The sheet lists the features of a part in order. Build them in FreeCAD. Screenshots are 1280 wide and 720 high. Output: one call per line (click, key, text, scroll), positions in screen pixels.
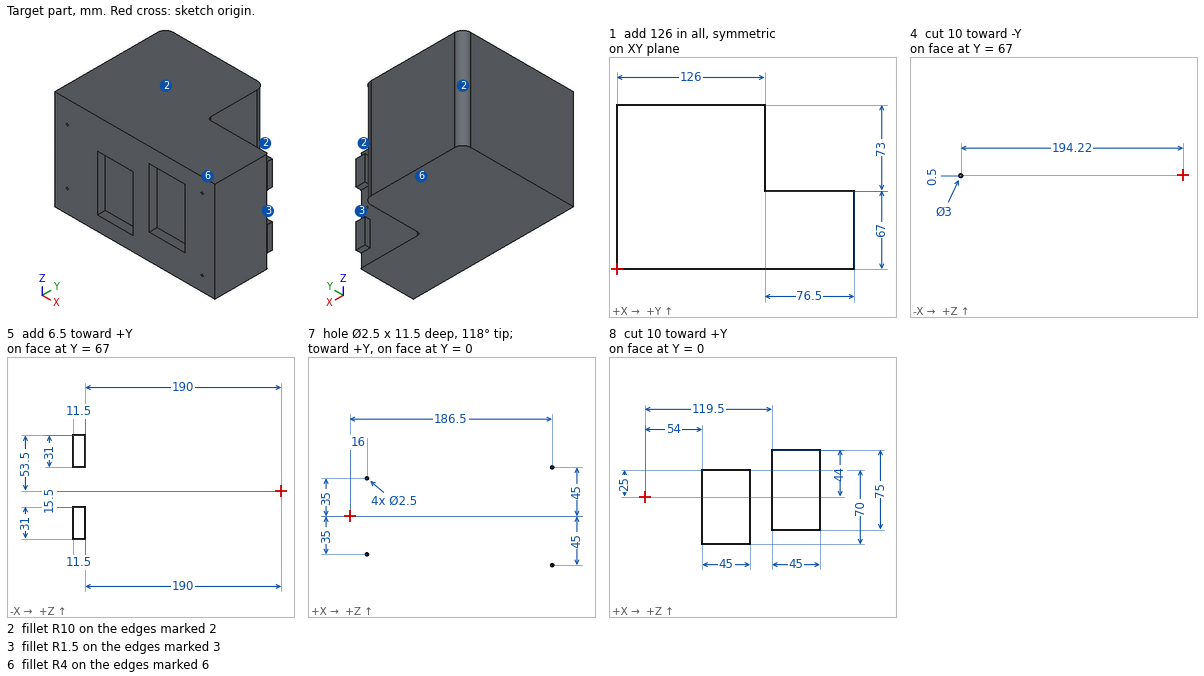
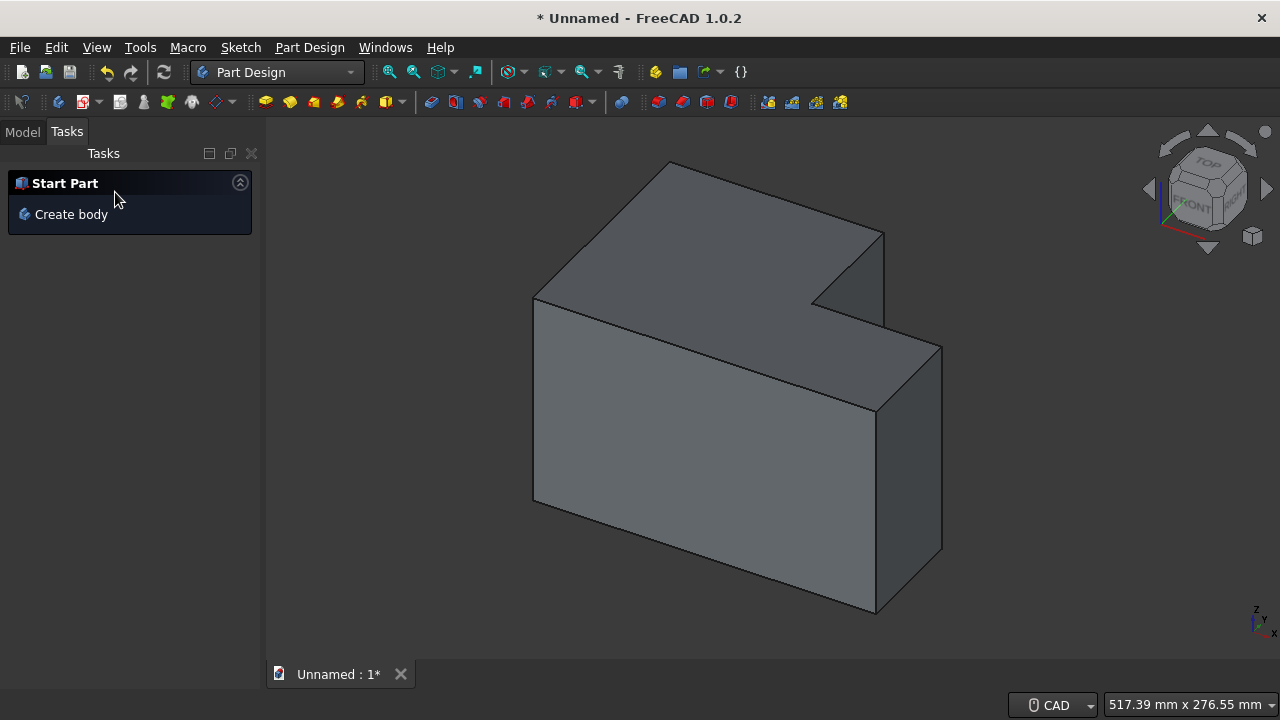
key(0)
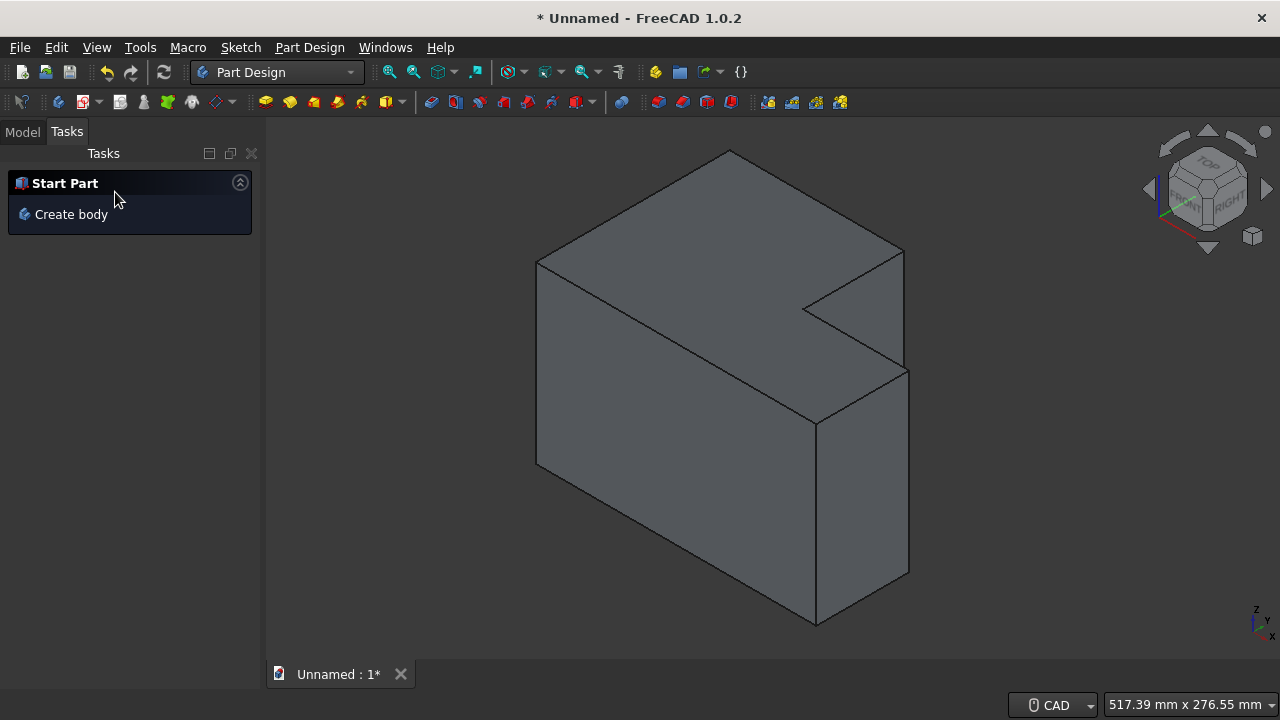
key(2)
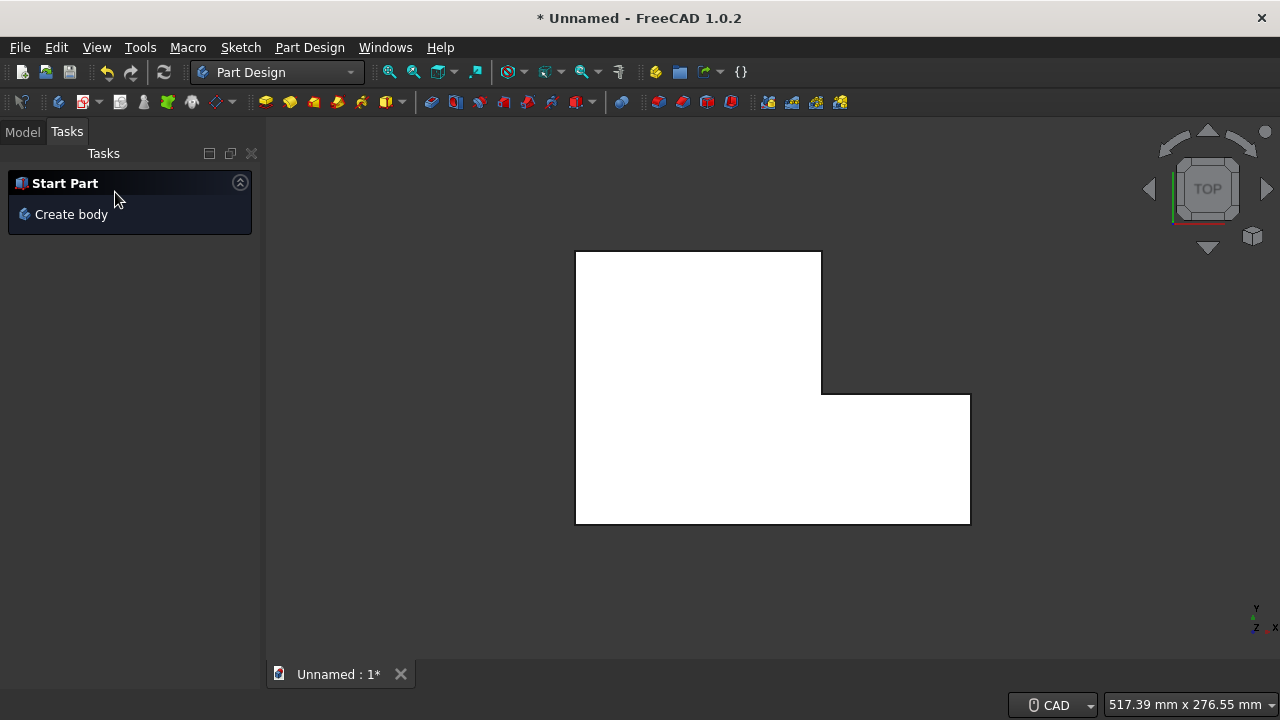
key(1)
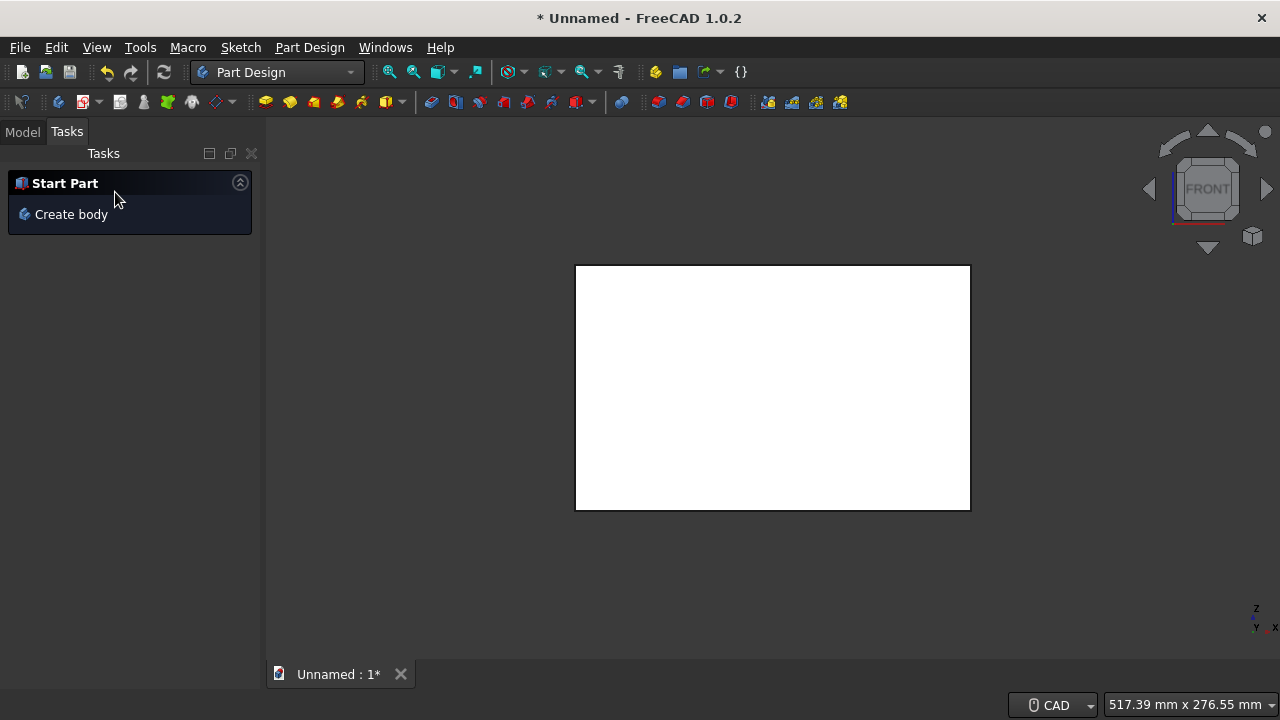
key(3)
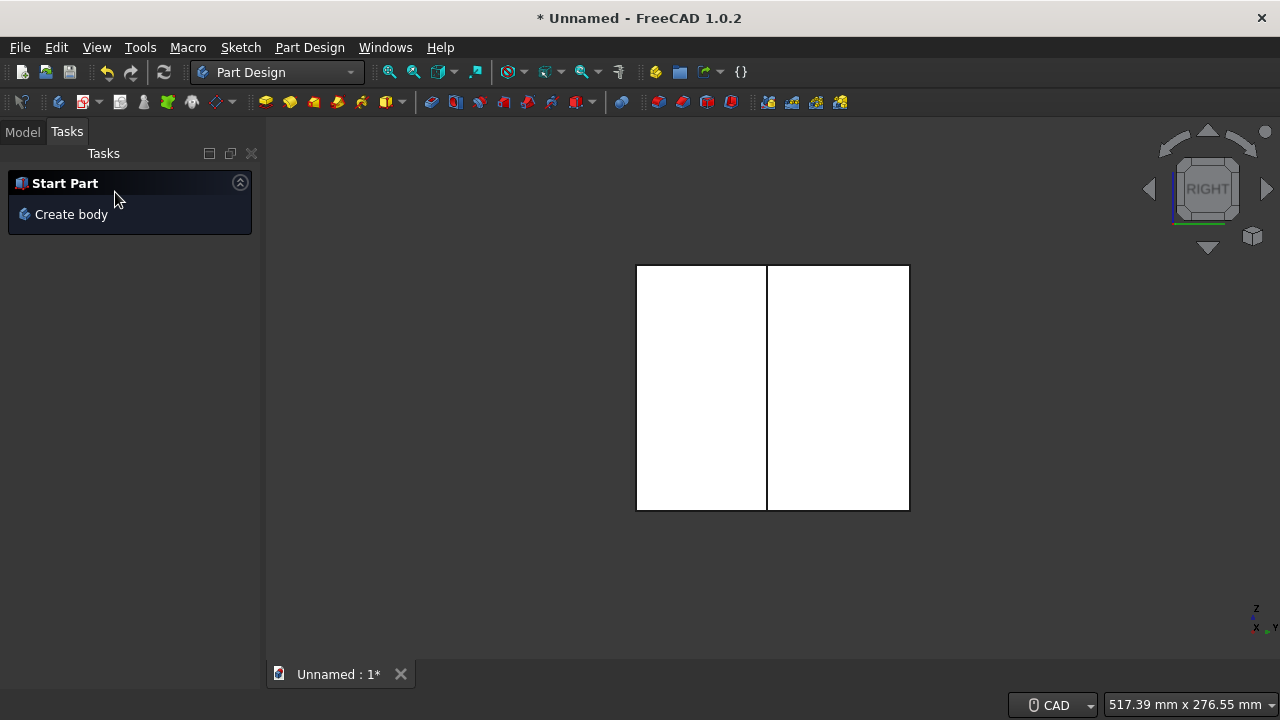
click(910, 387)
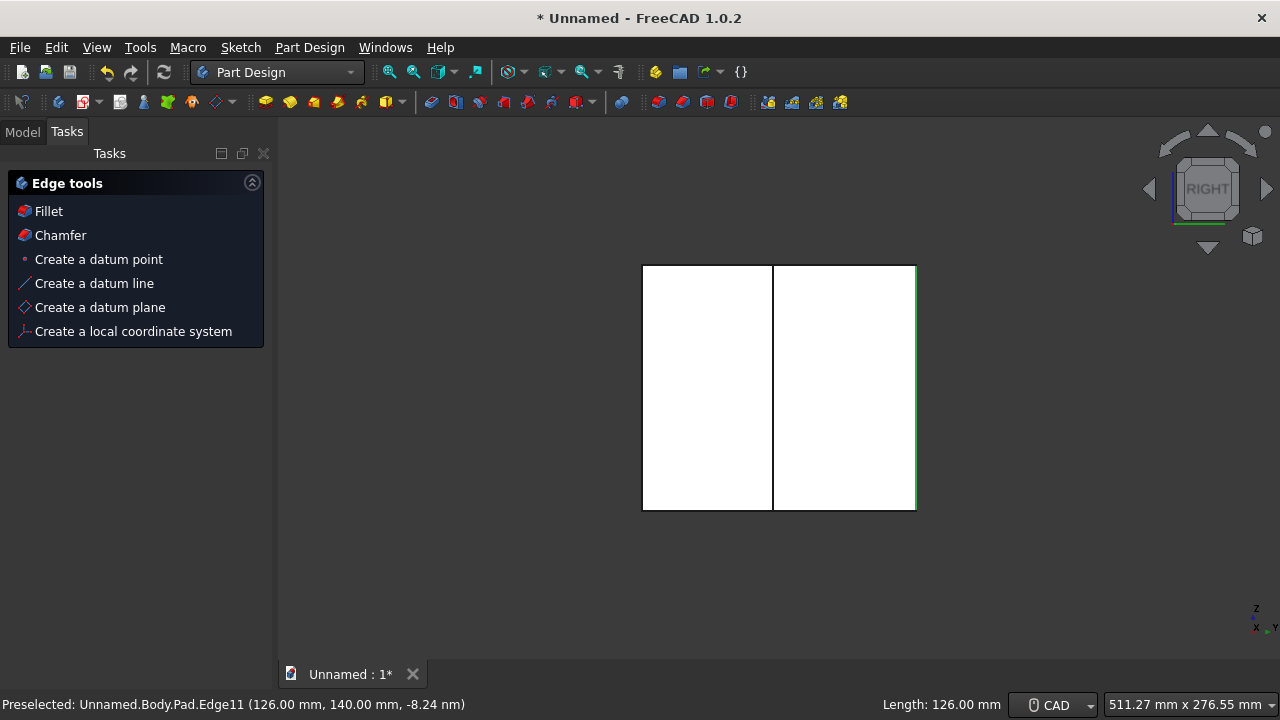
key(5)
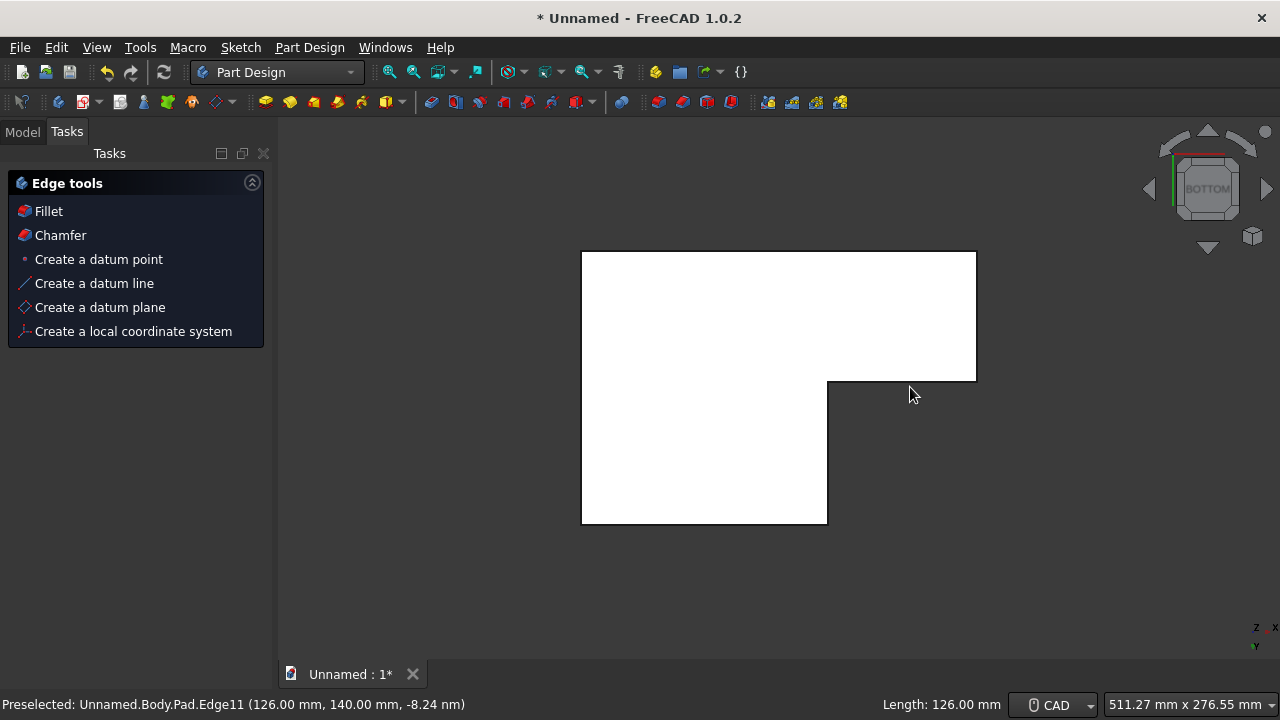
key(4)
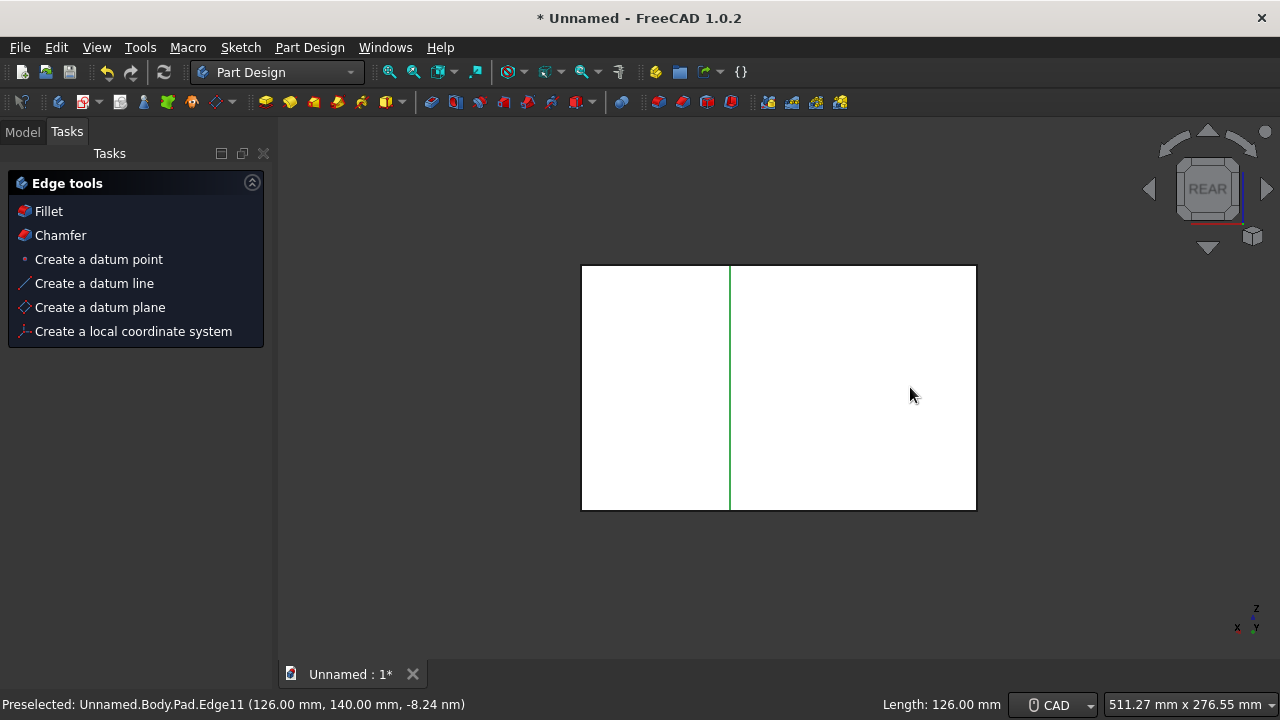
click(977, 387, ctrl)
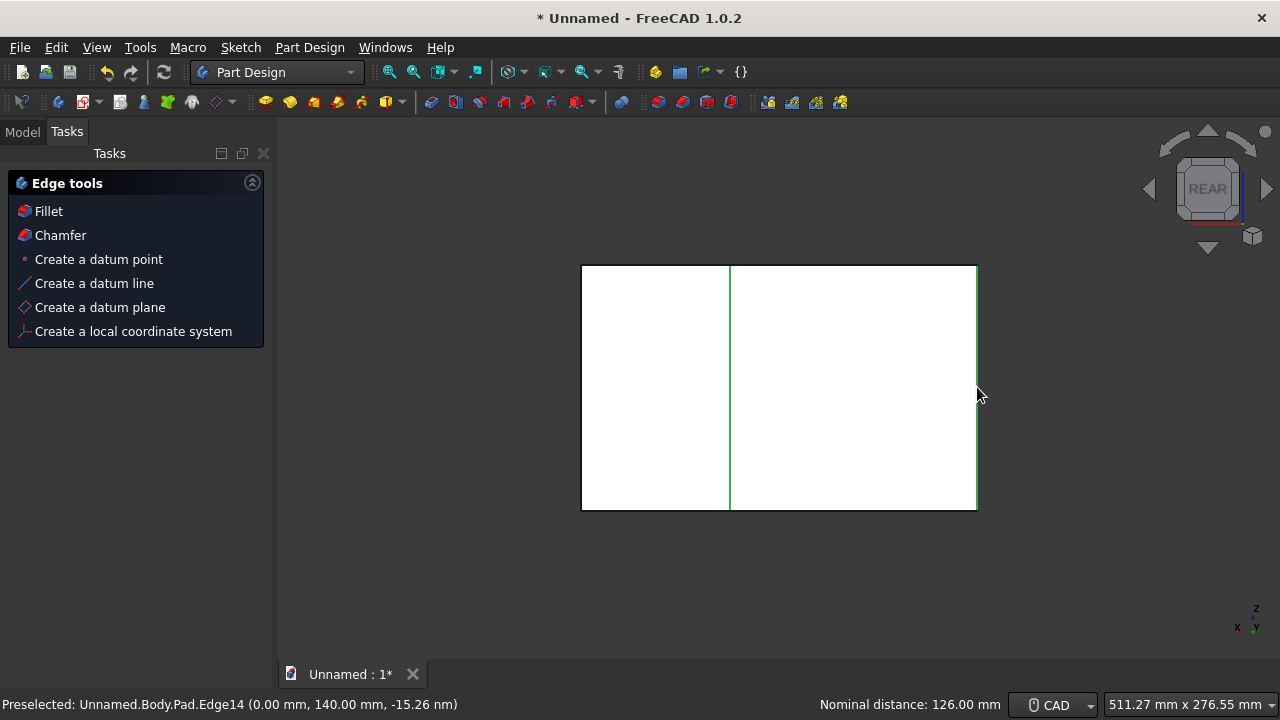
click(660, 102)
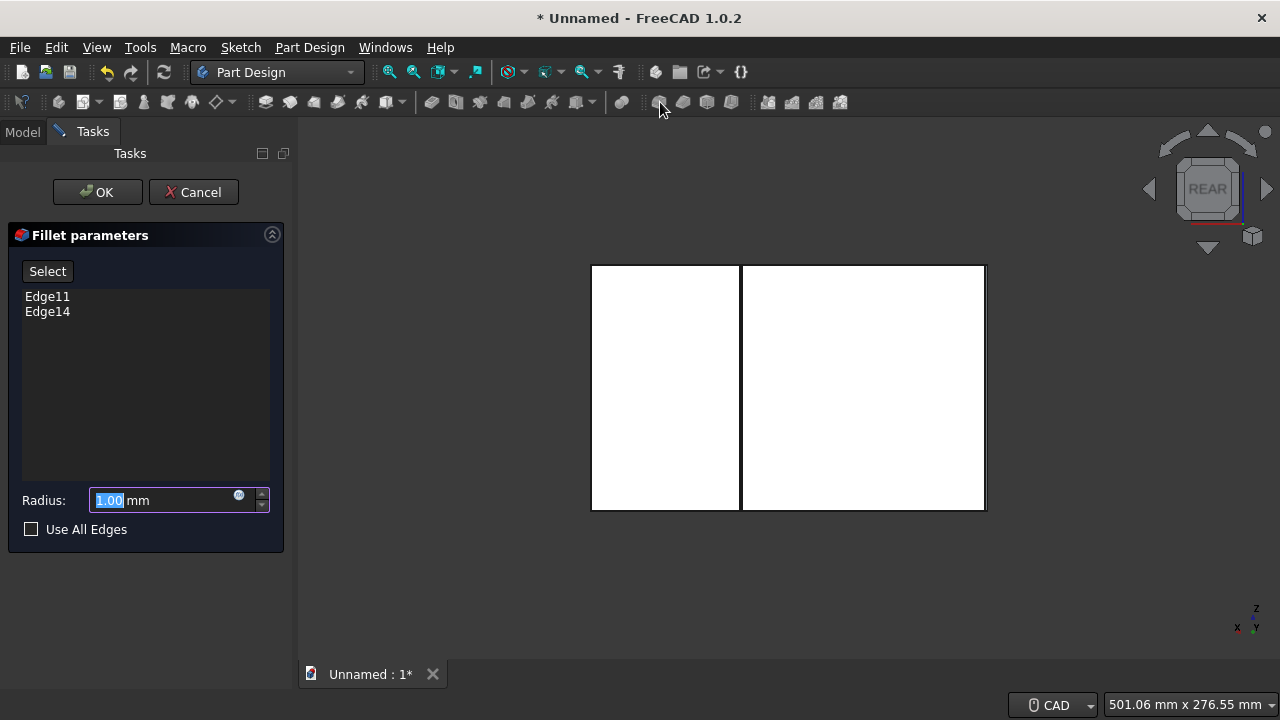
text(10)
key(Tab)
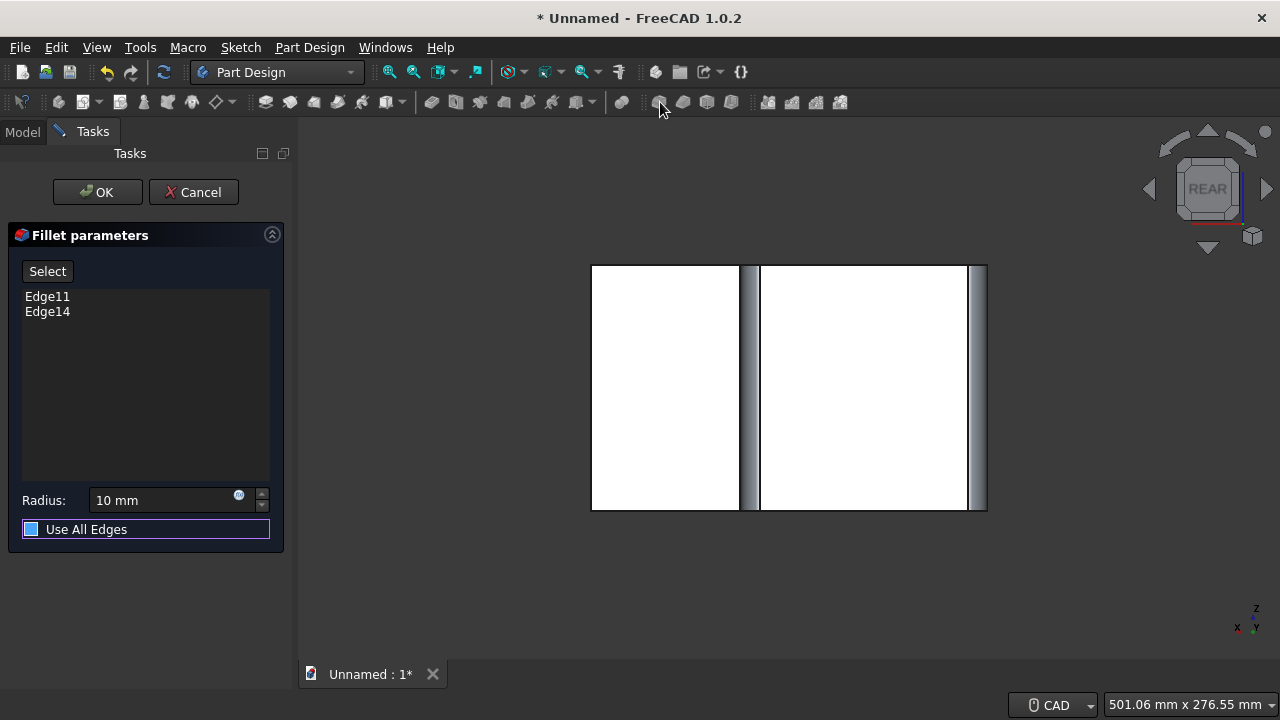
click(98, 192)